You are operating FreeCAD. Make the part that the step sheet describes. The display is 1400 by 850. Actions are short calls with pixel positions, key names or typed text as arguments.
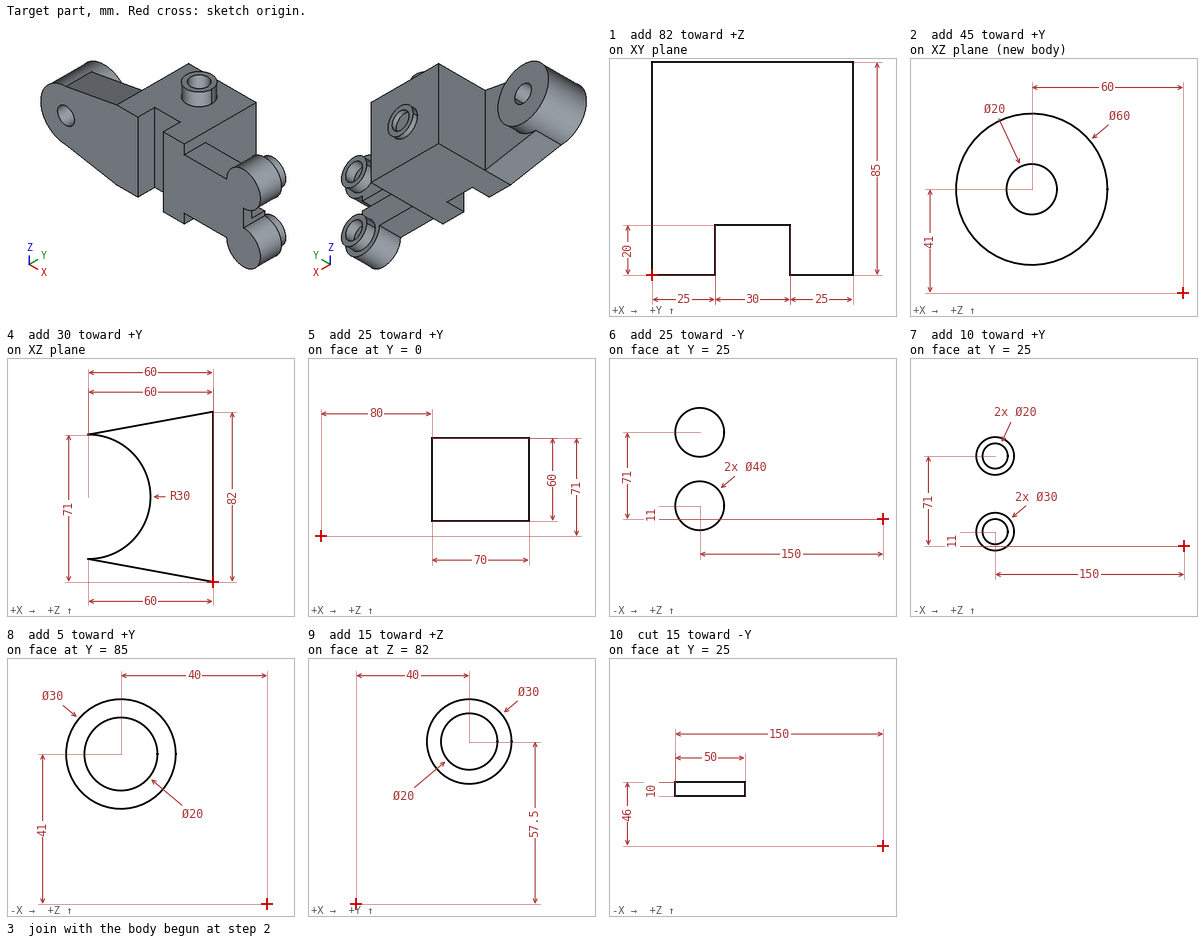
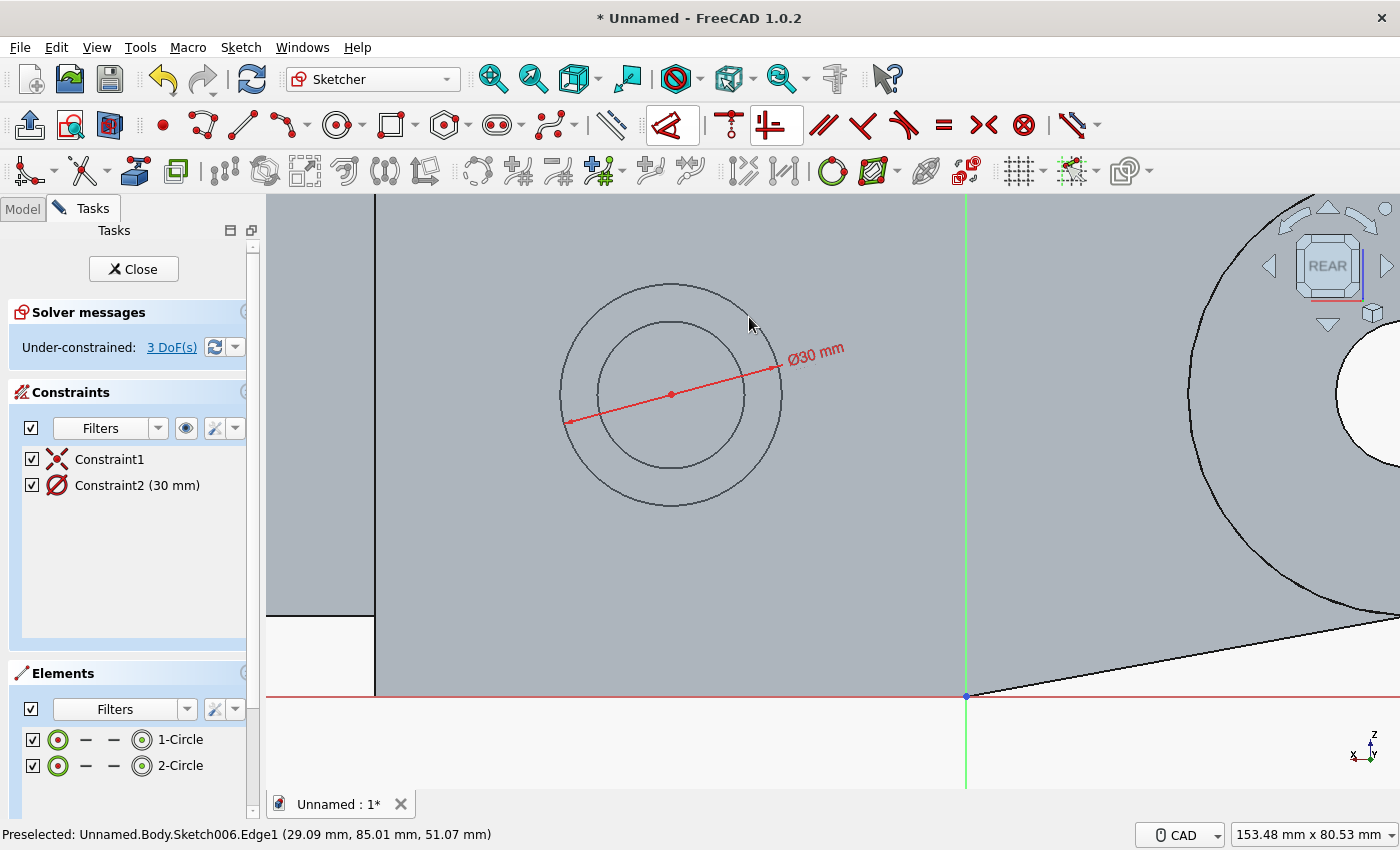
click(723, 343)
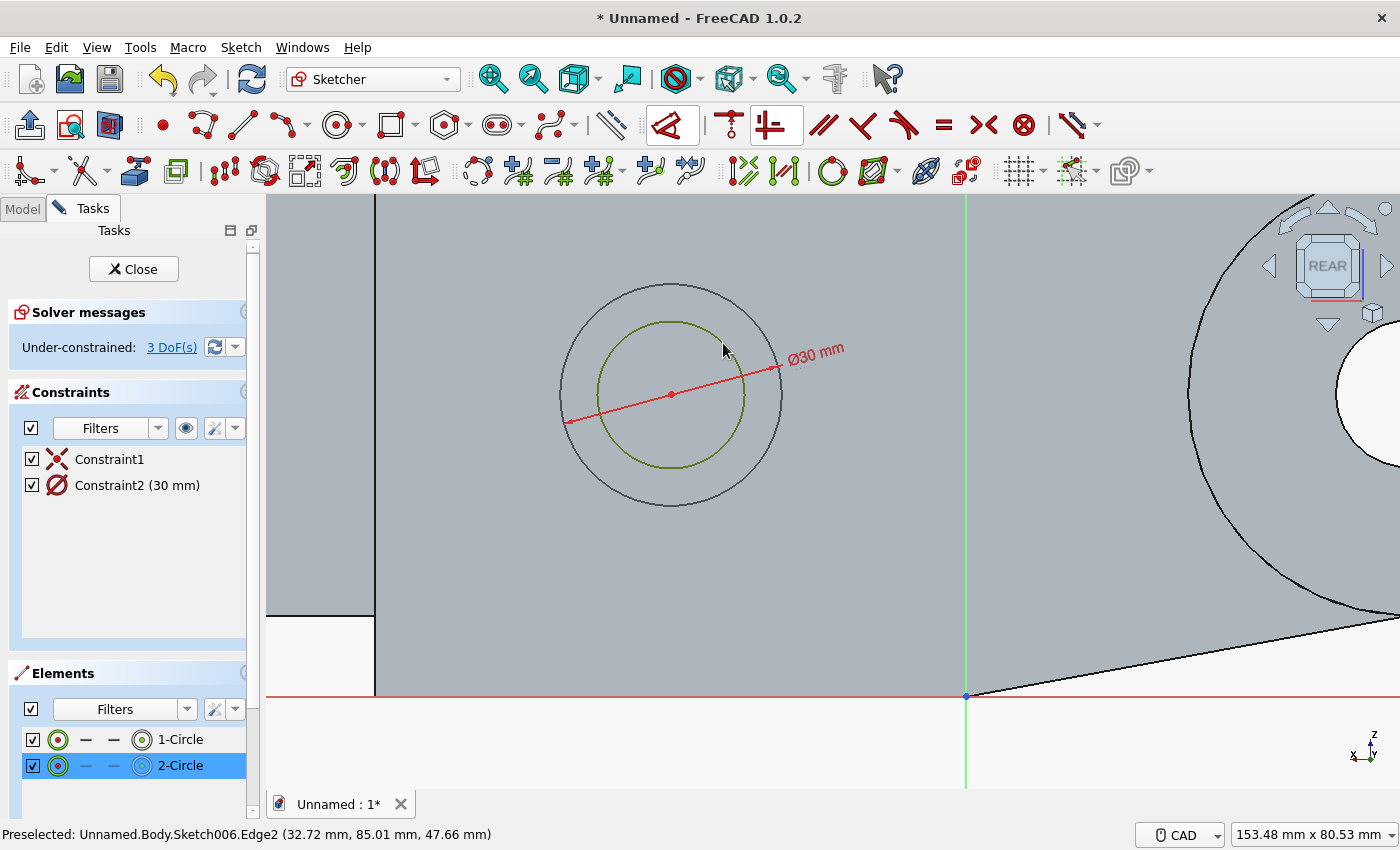
key(k)
key(o)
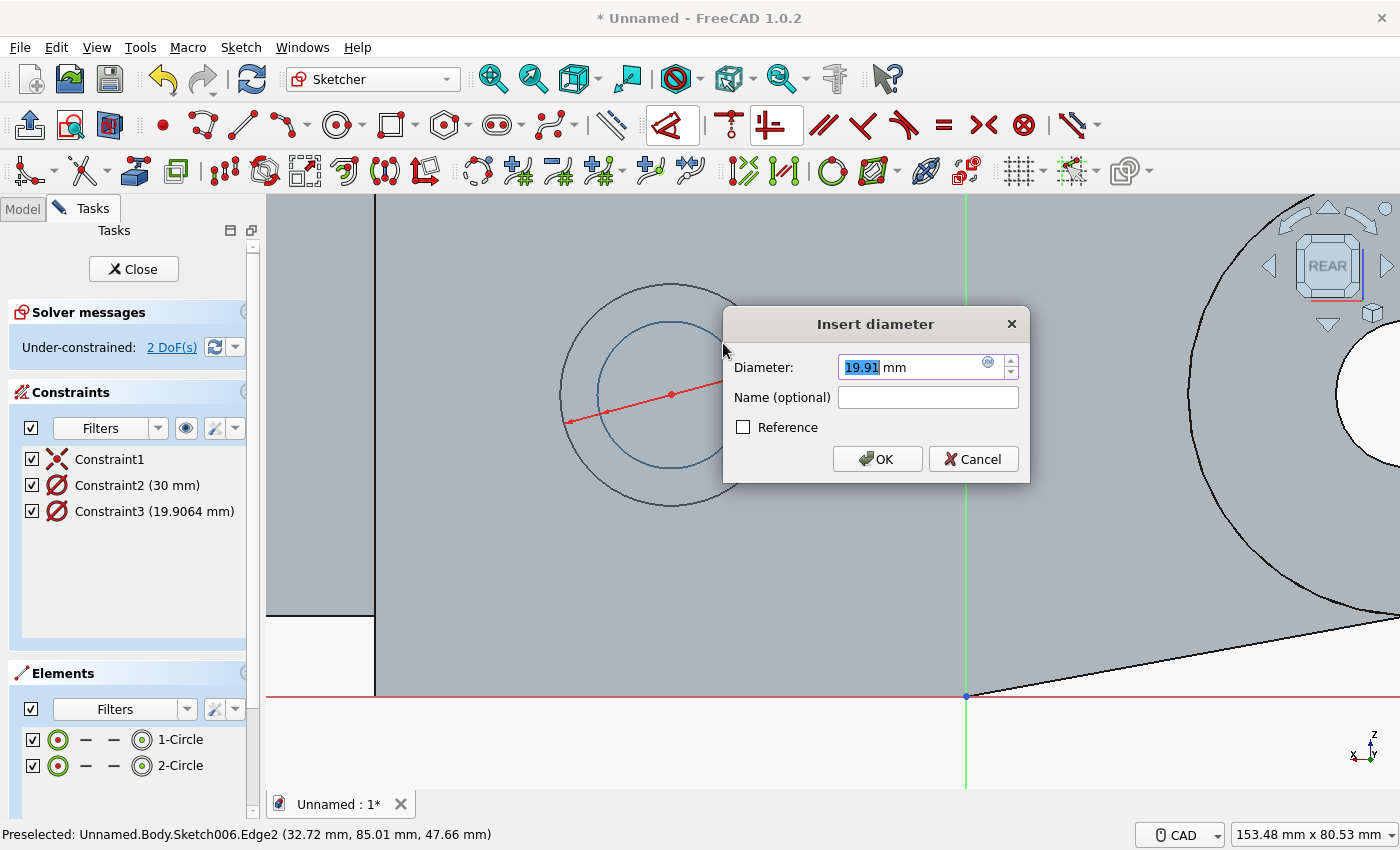
text(20)
key(Return)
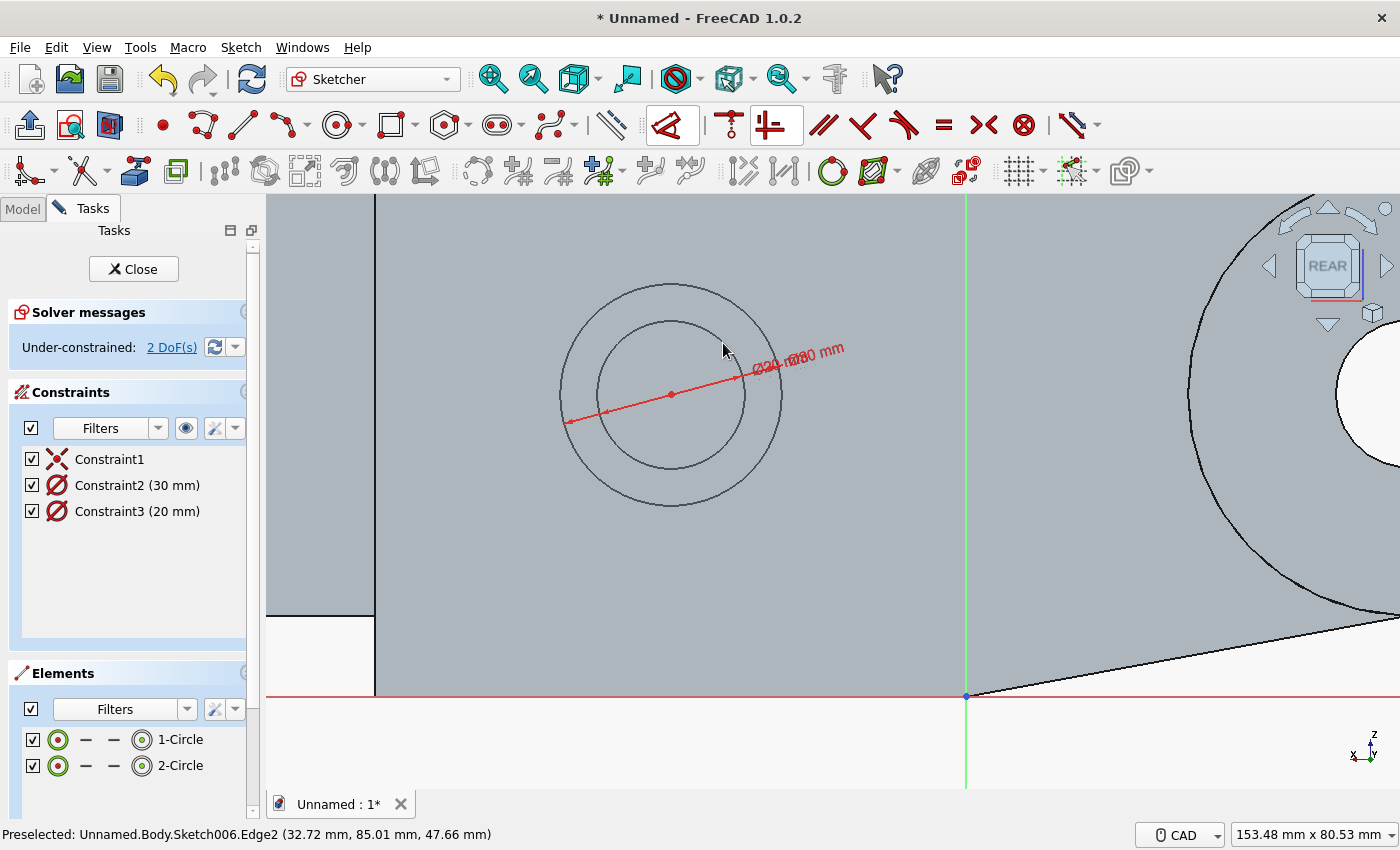
click(671, 395)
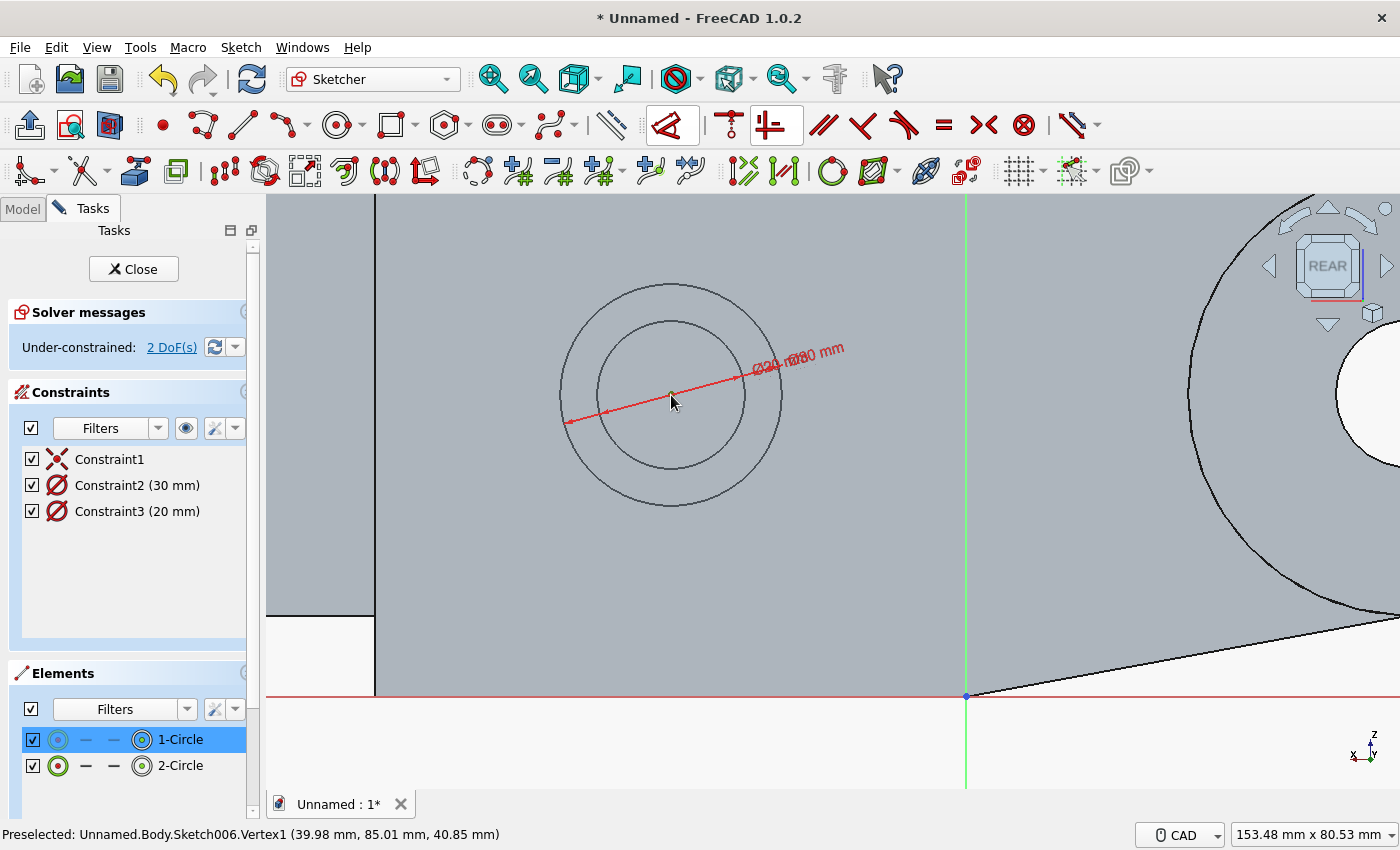
click(694, 126)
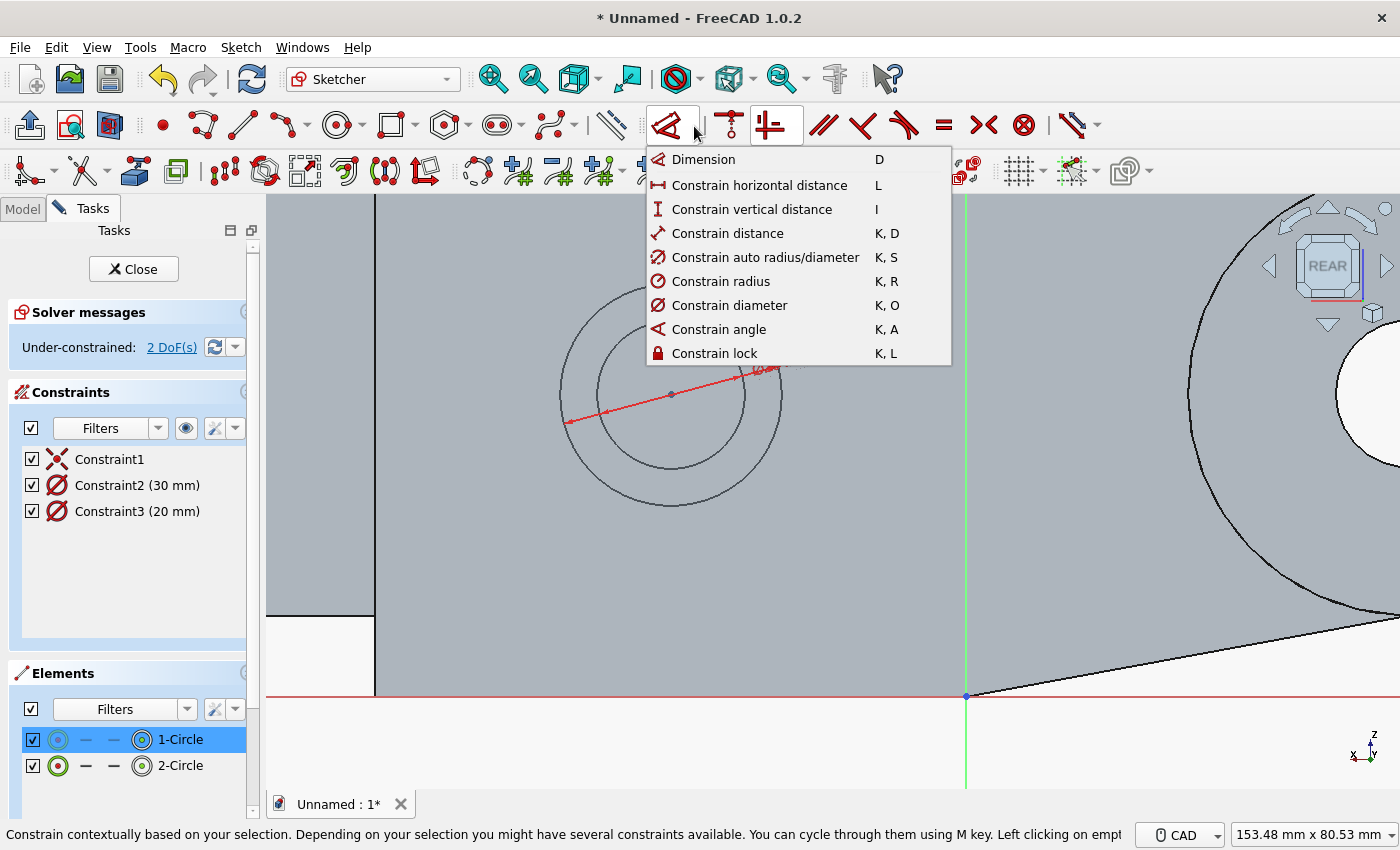
click(799, 185)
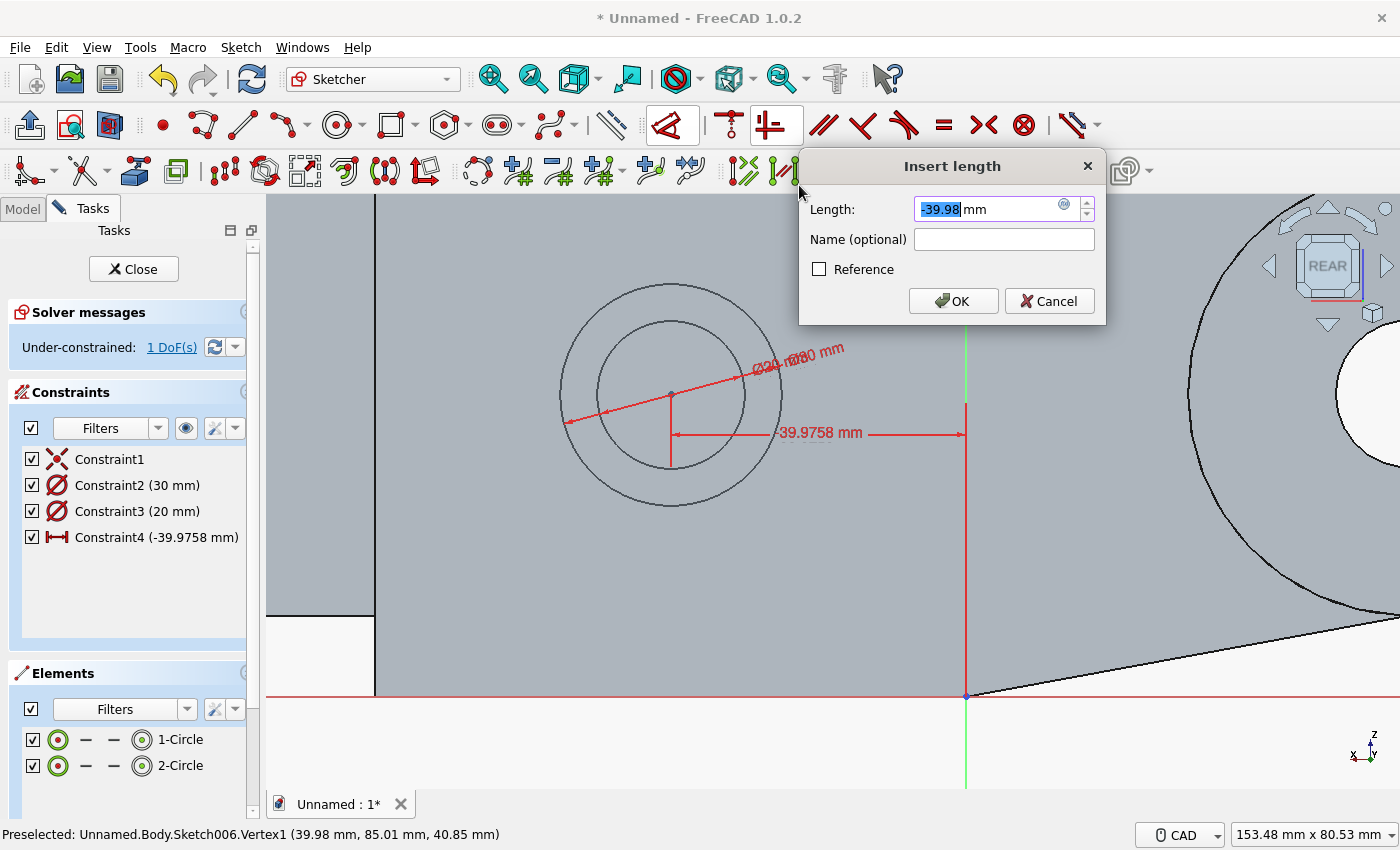
text(-40)
key(Return)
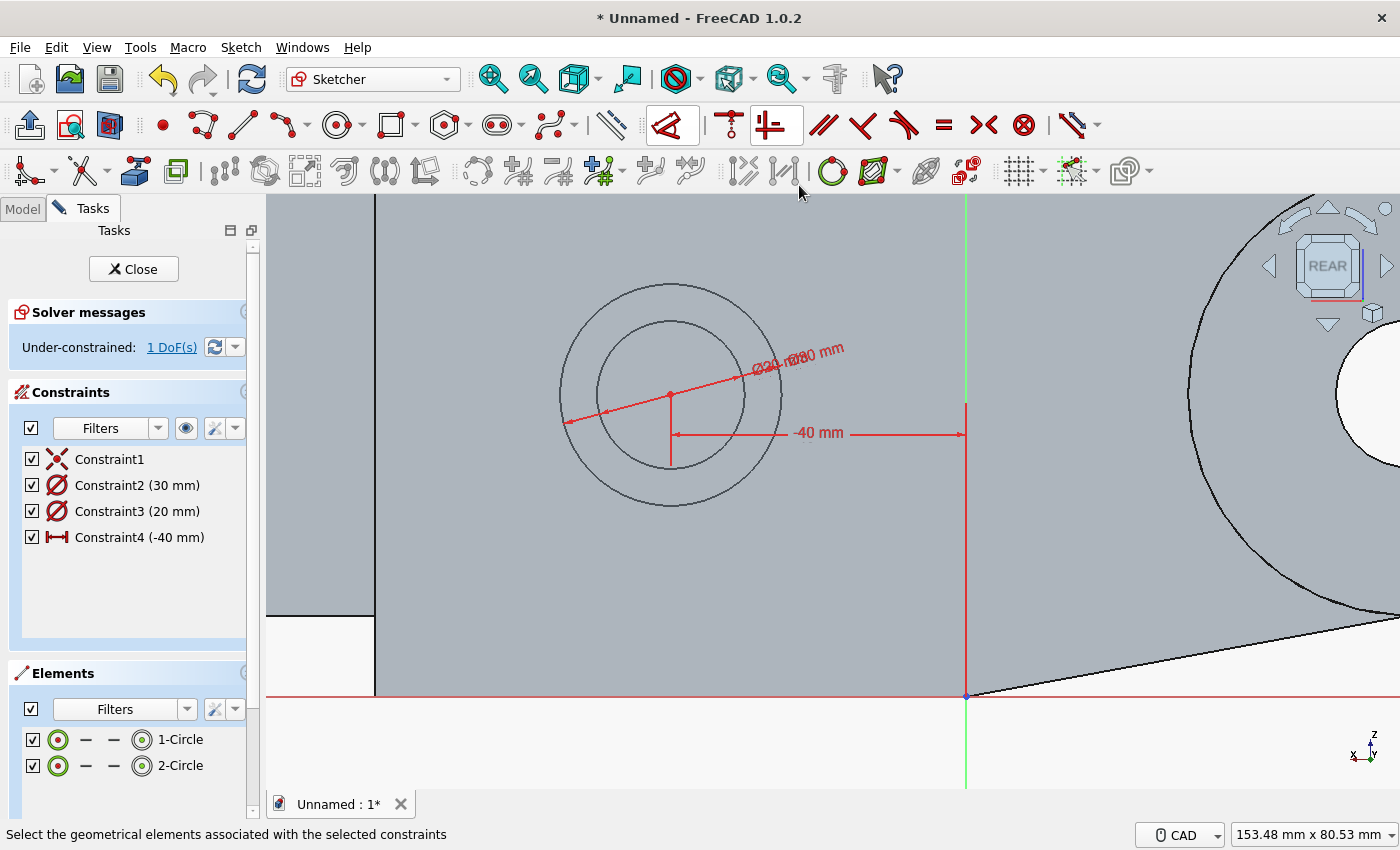
click(671, 395)